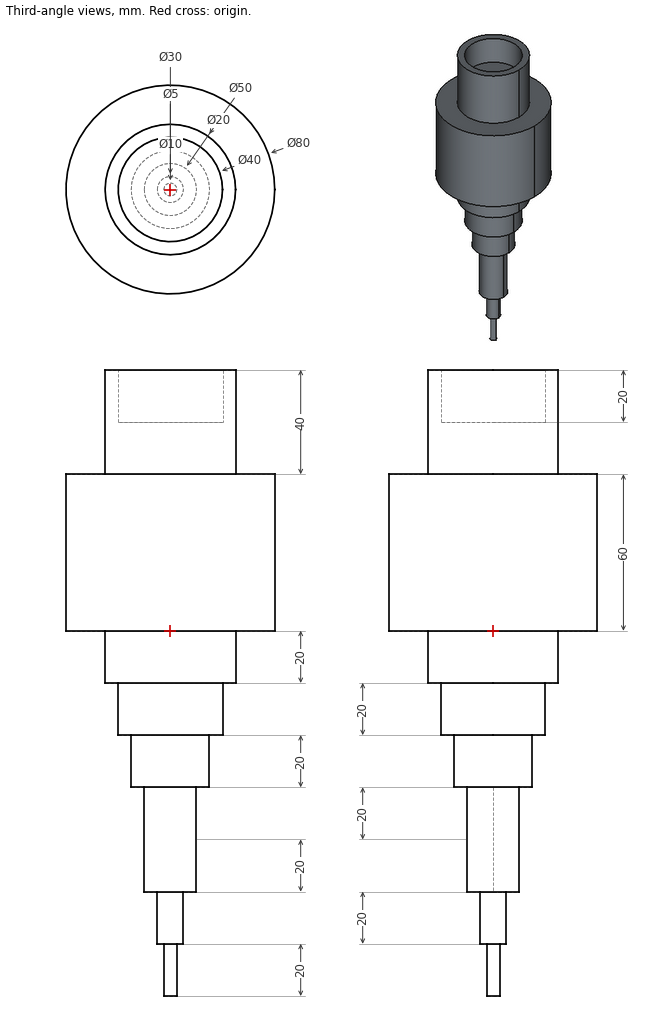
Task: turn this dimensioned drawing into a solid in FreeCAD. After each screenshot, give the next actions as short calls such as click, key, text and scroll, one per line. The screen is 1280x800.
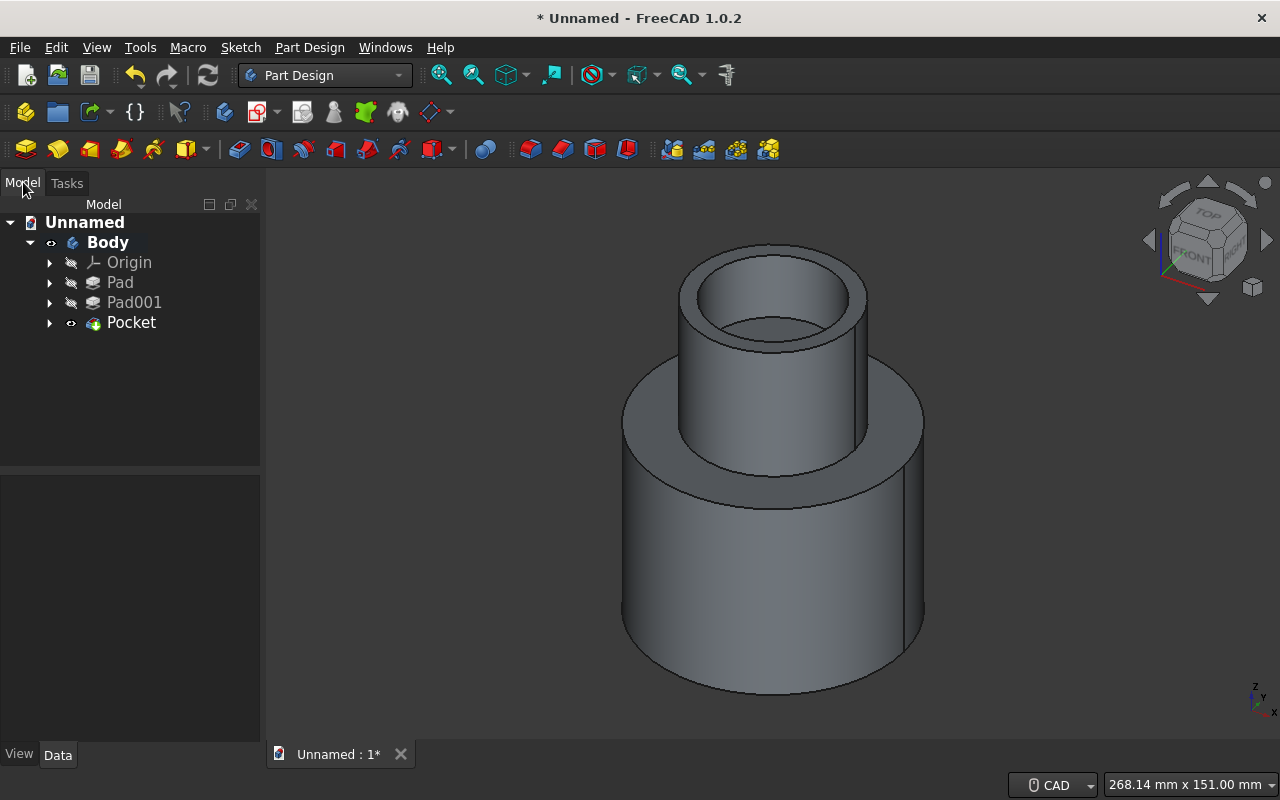
click(50, 263)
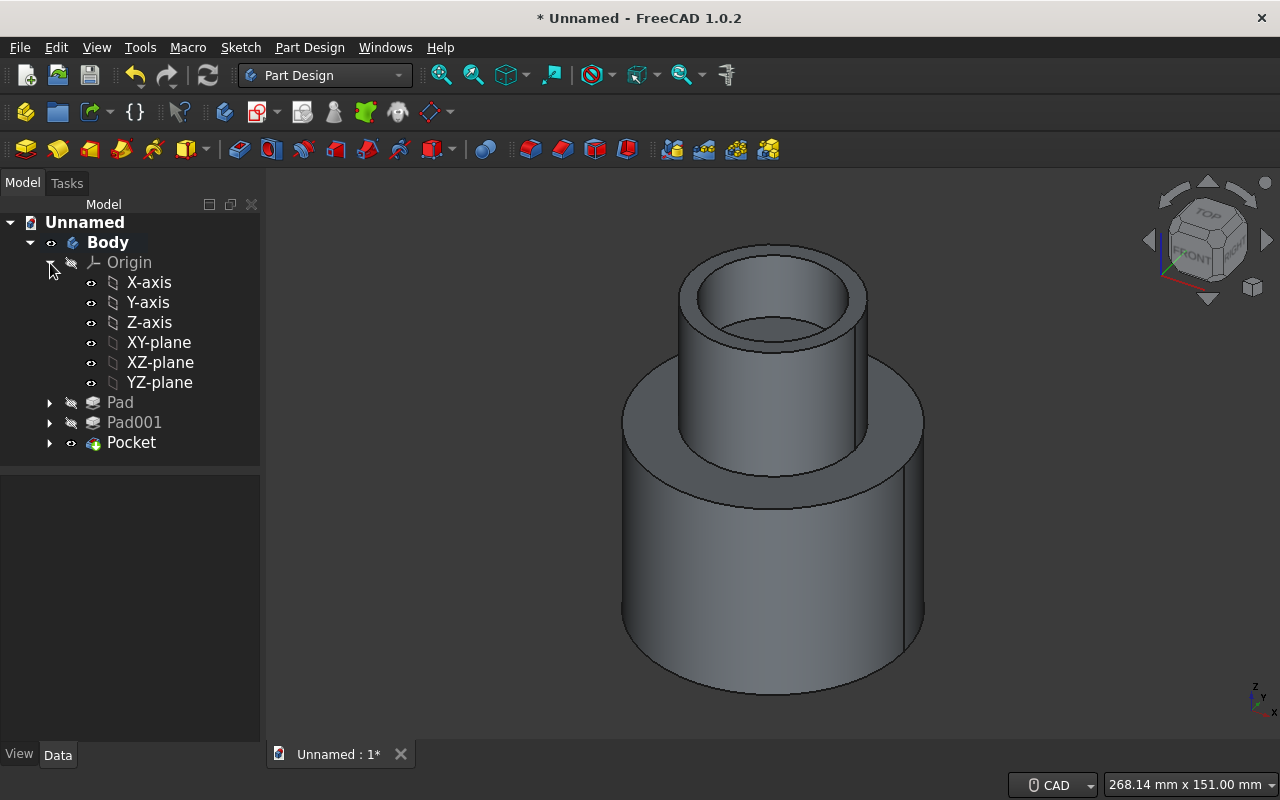
click(136, 343)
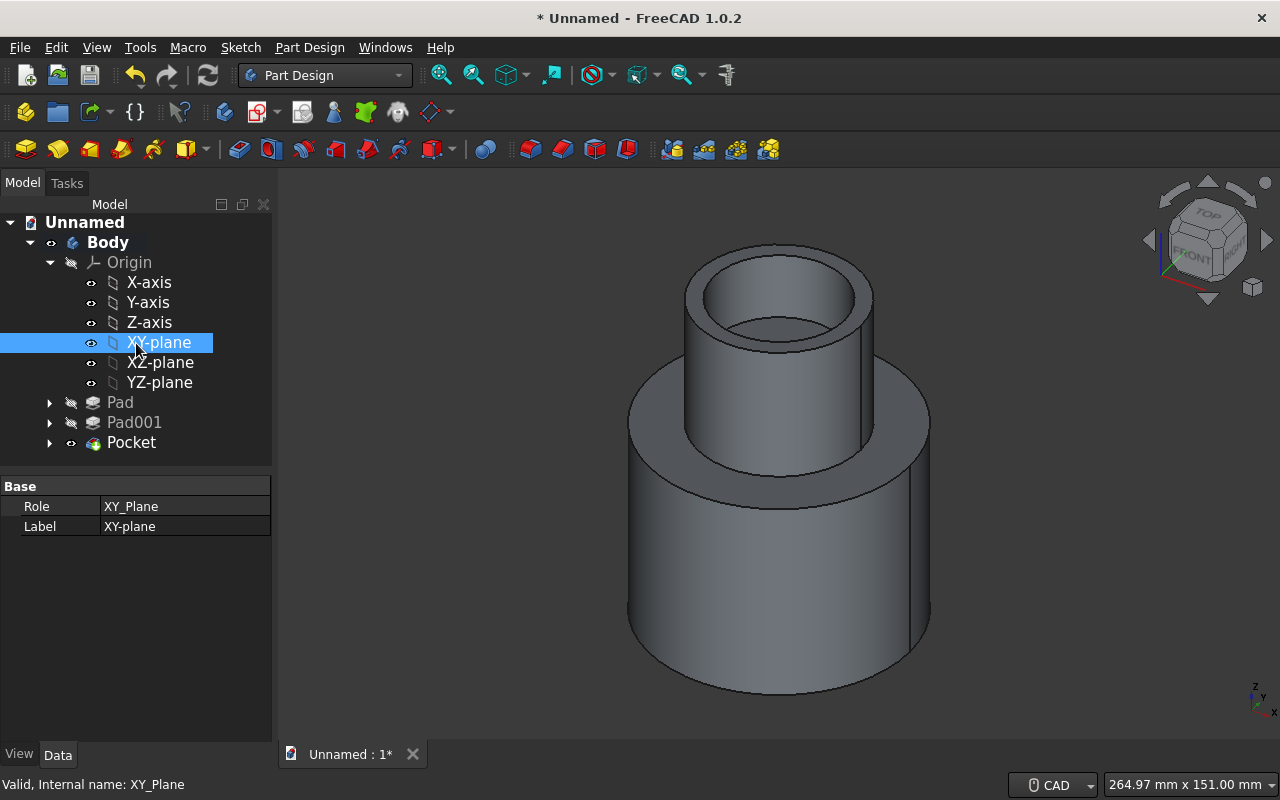
click(430, 112)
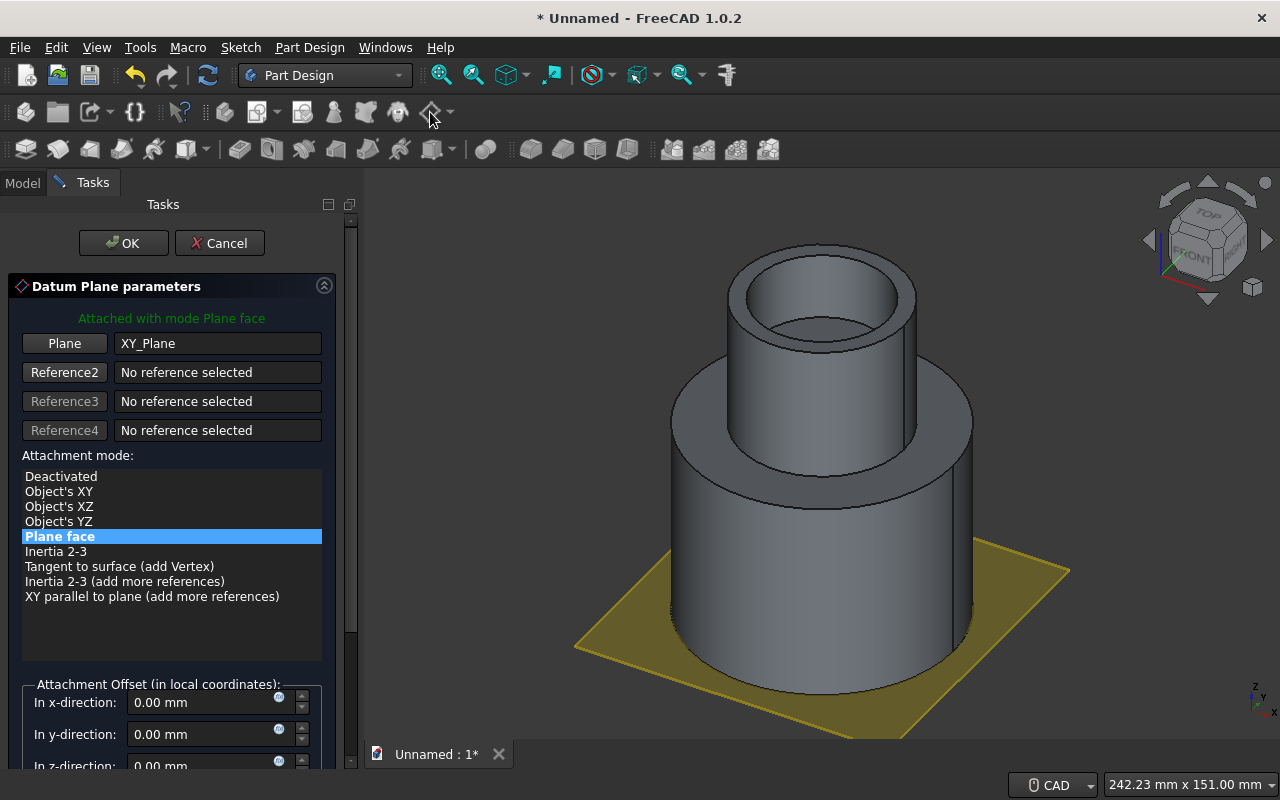
scroll(351, 491, down, 2)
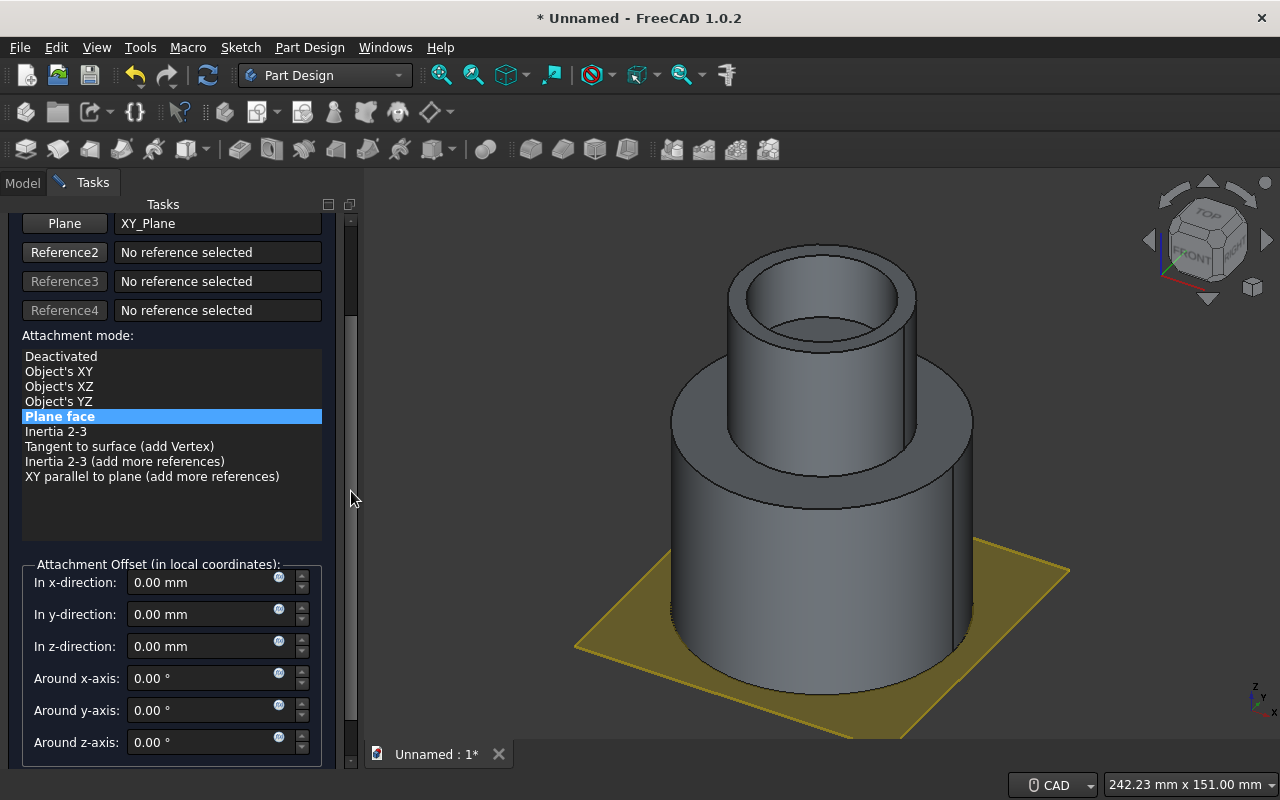
triple_click(210, 646)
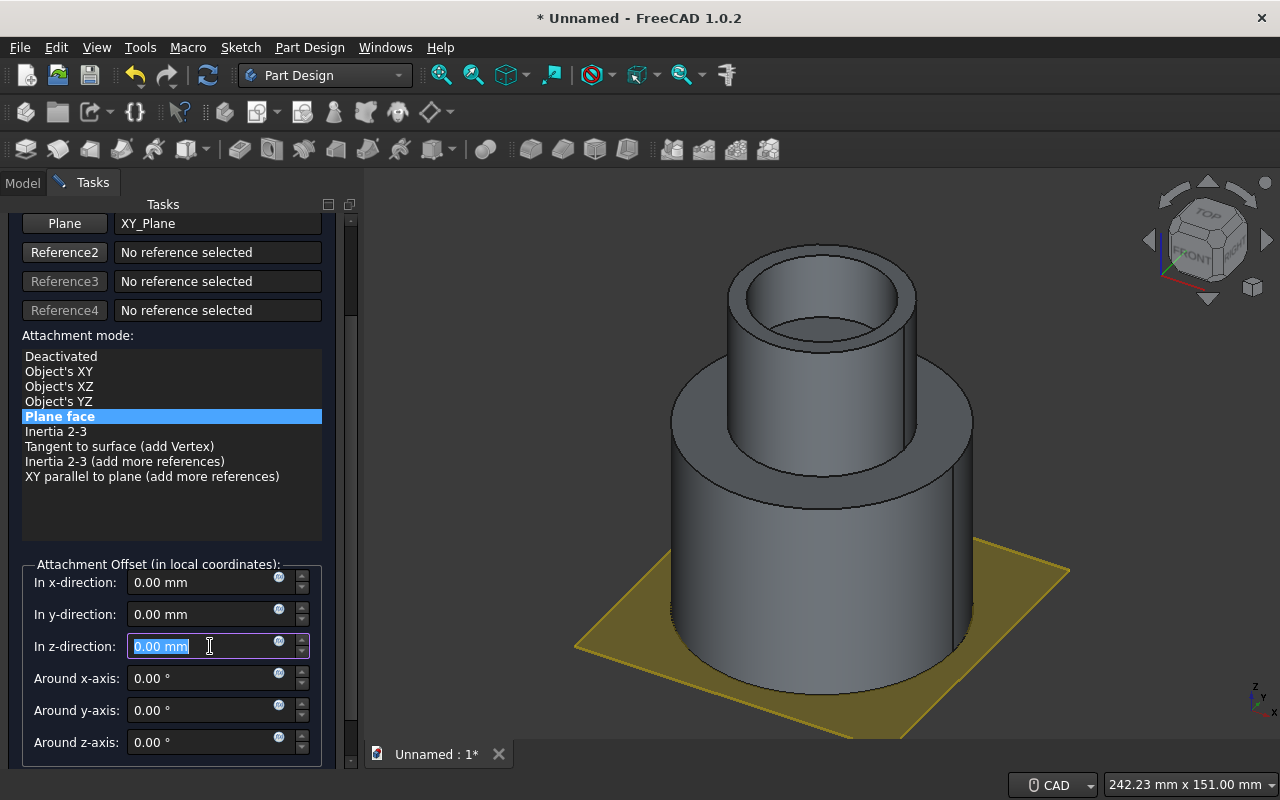
text(-20)
key(Tab)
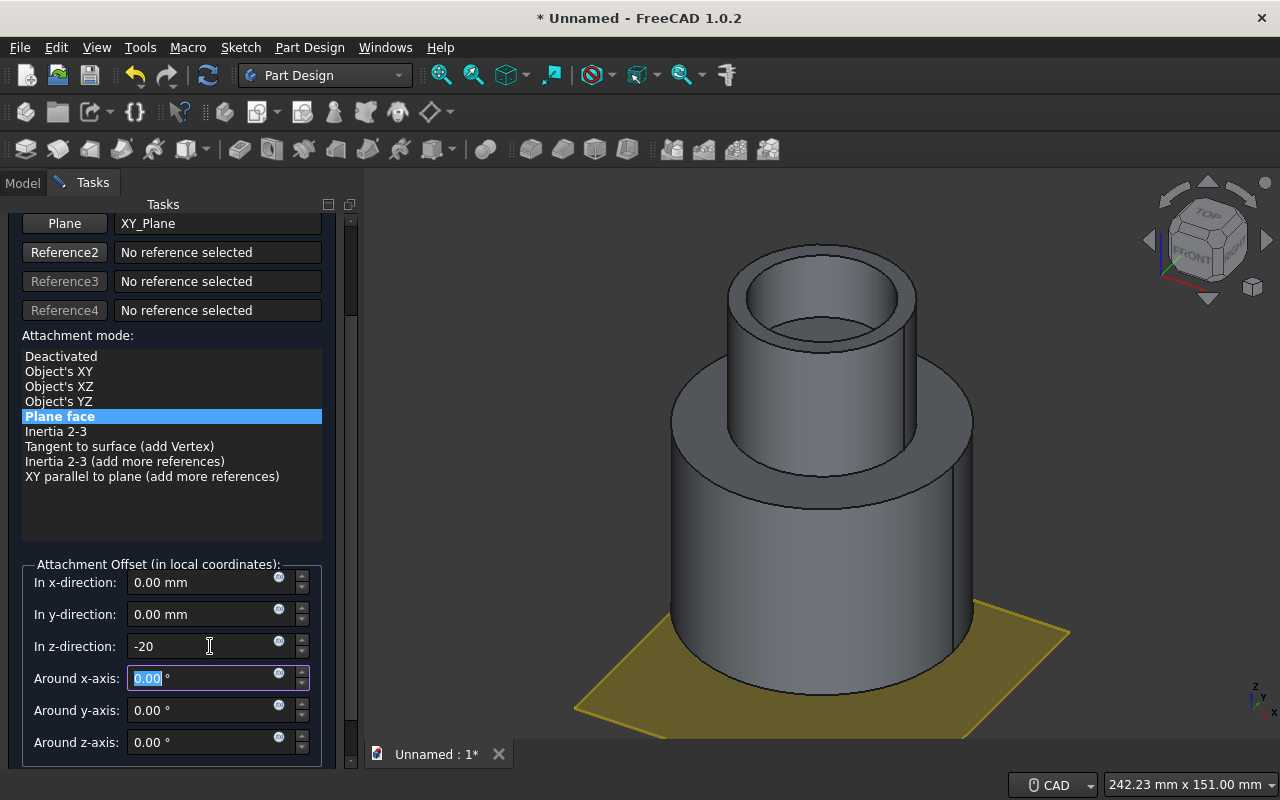
scroll(351, 491, up, 3)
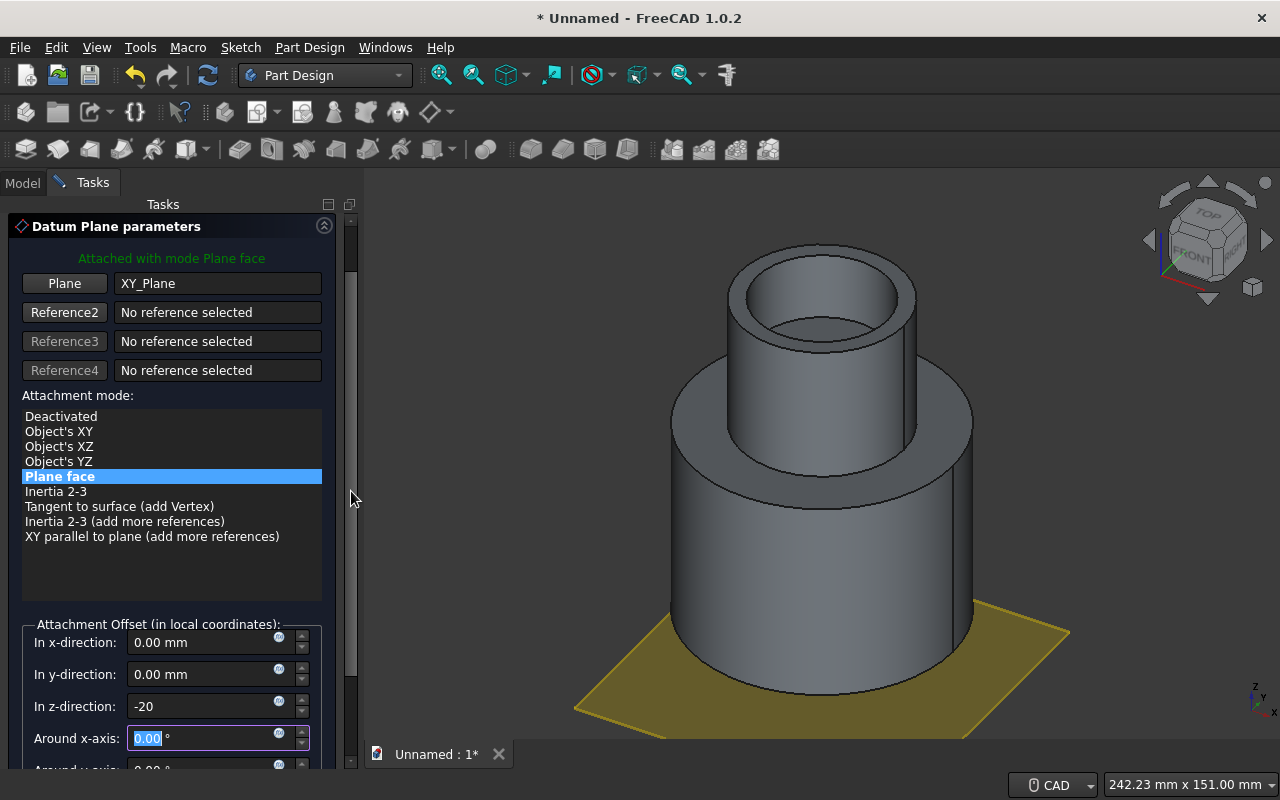
click(124, 243)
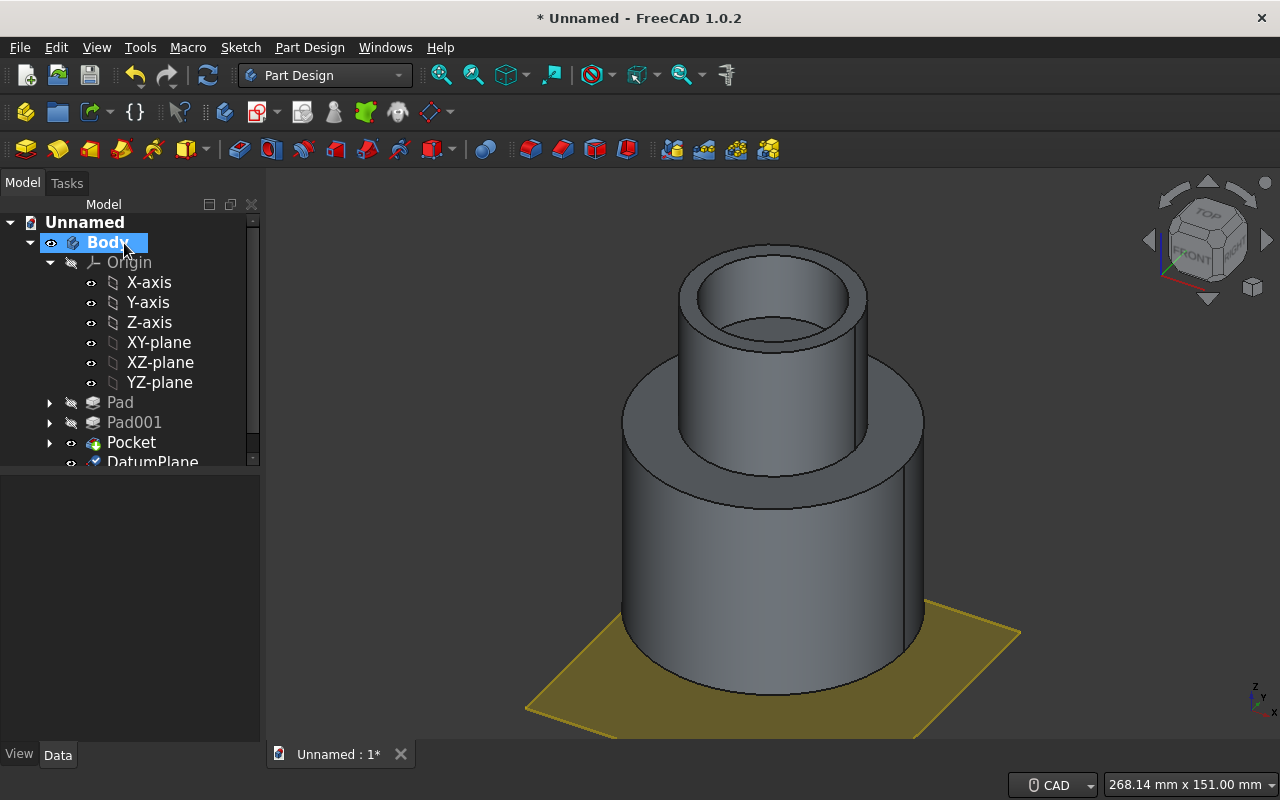
click(116, 463)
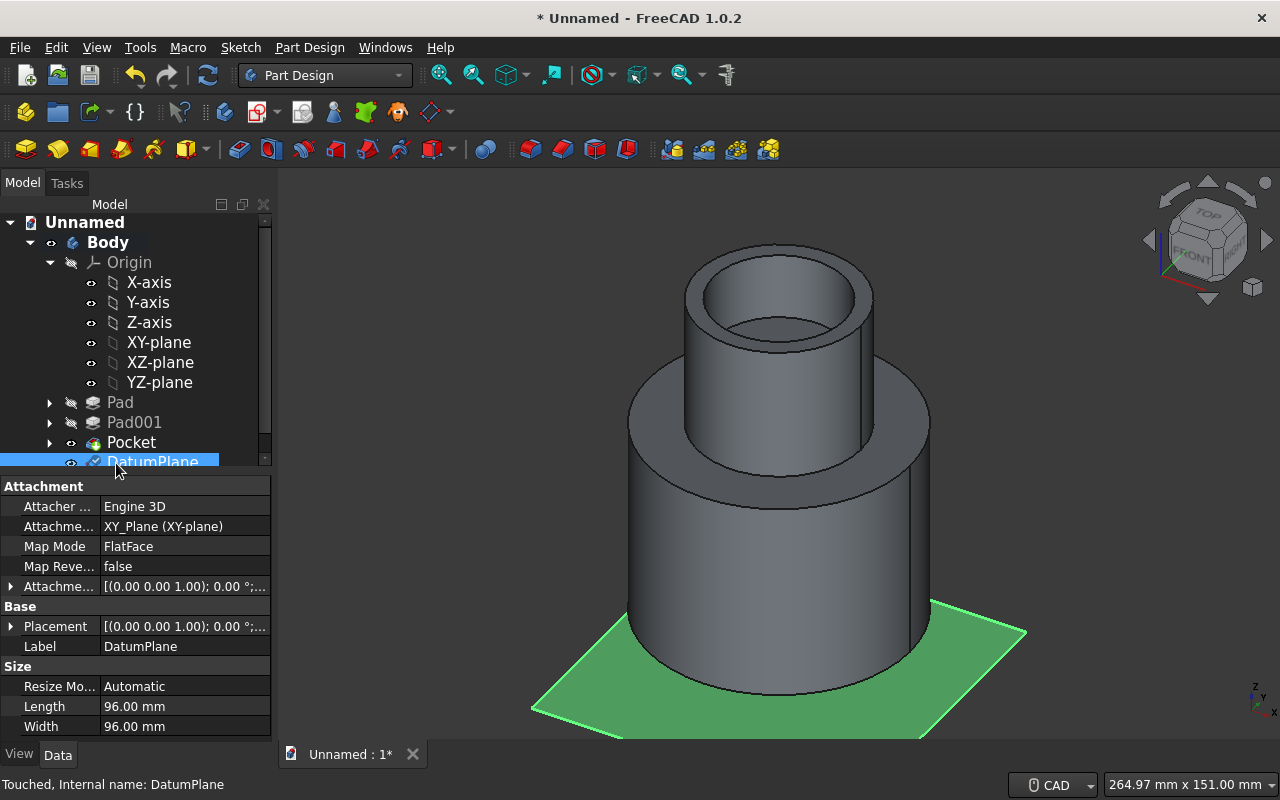
click(258, 112)